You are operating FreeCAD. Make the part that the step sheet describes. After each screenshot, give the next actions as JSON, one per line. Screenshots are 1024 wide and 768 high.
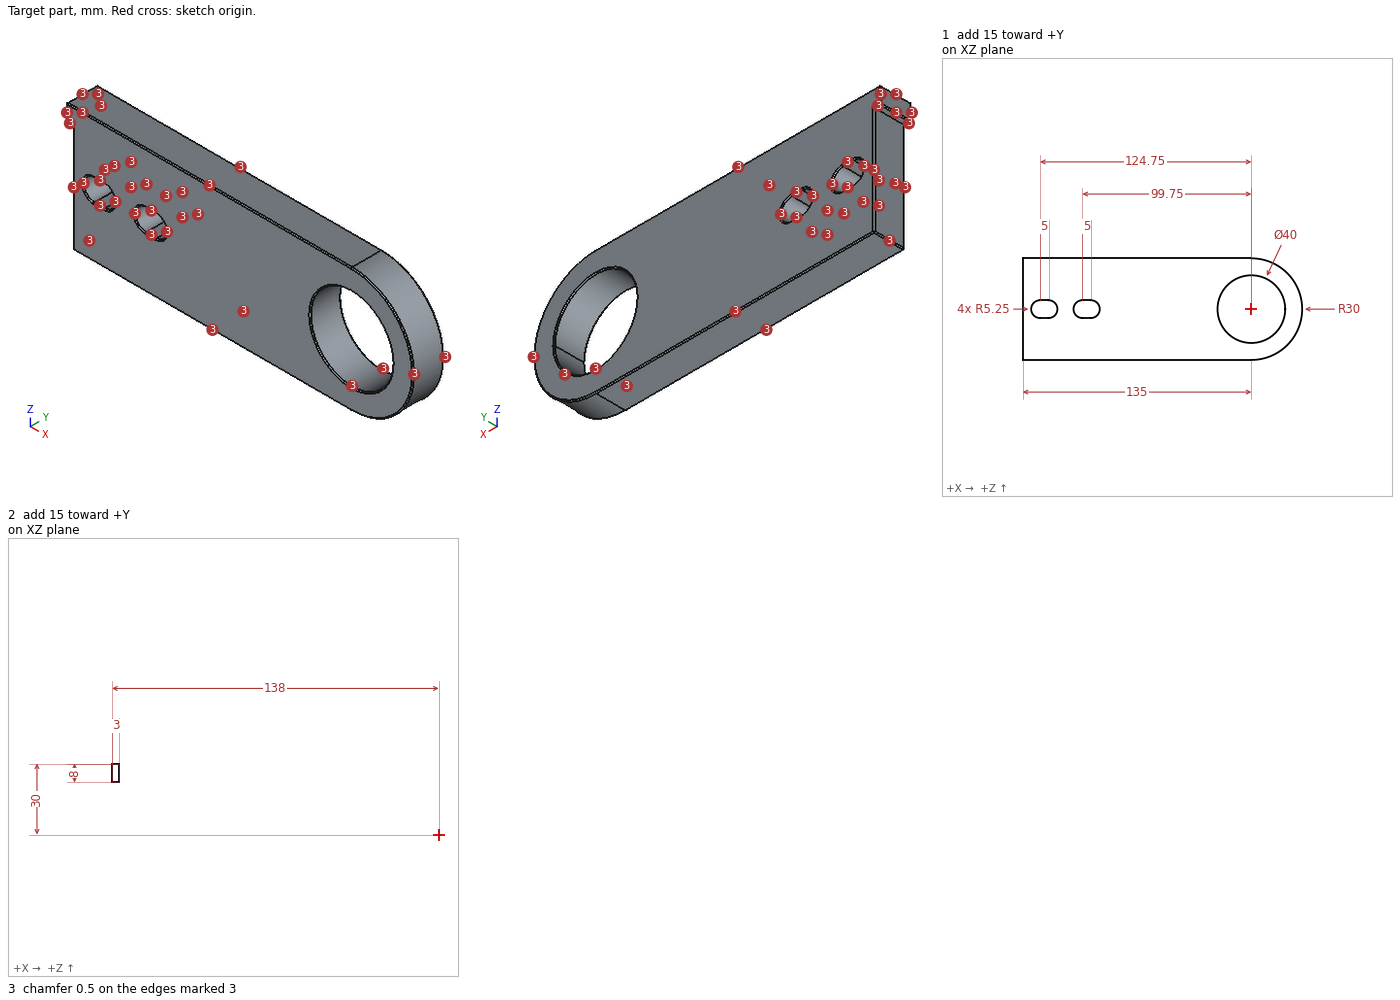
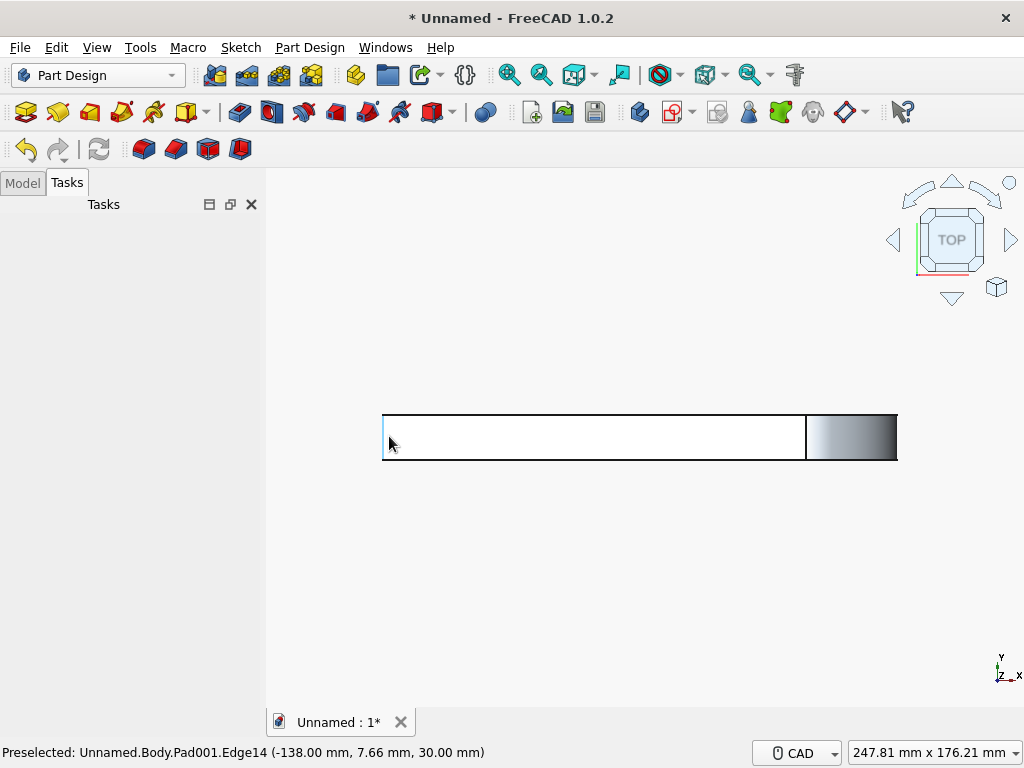
{"action": "key", "text": "1"}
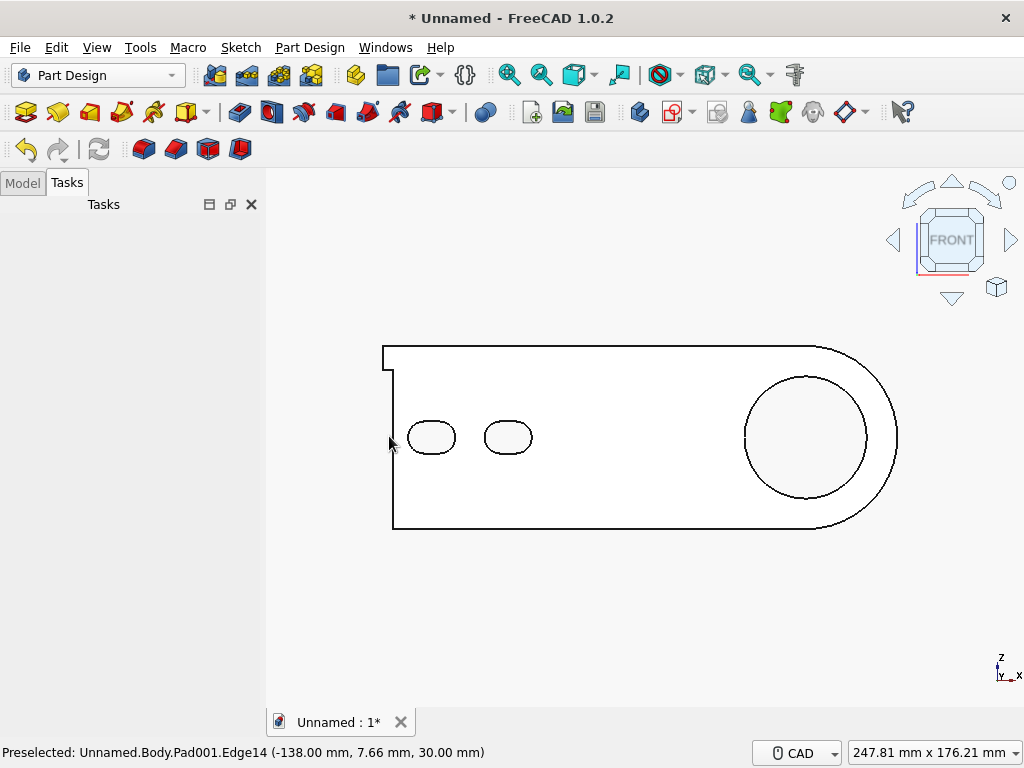
{"action": "key", "text": "3"}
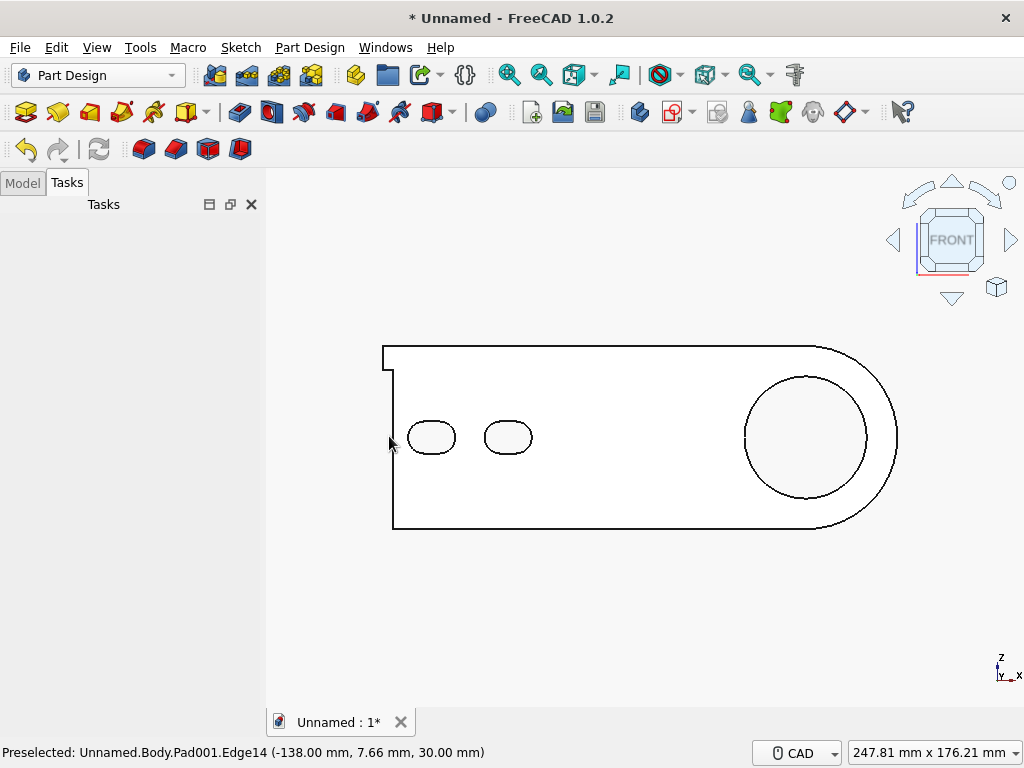
{"action": "left_click", "coordinate": [510, 76]}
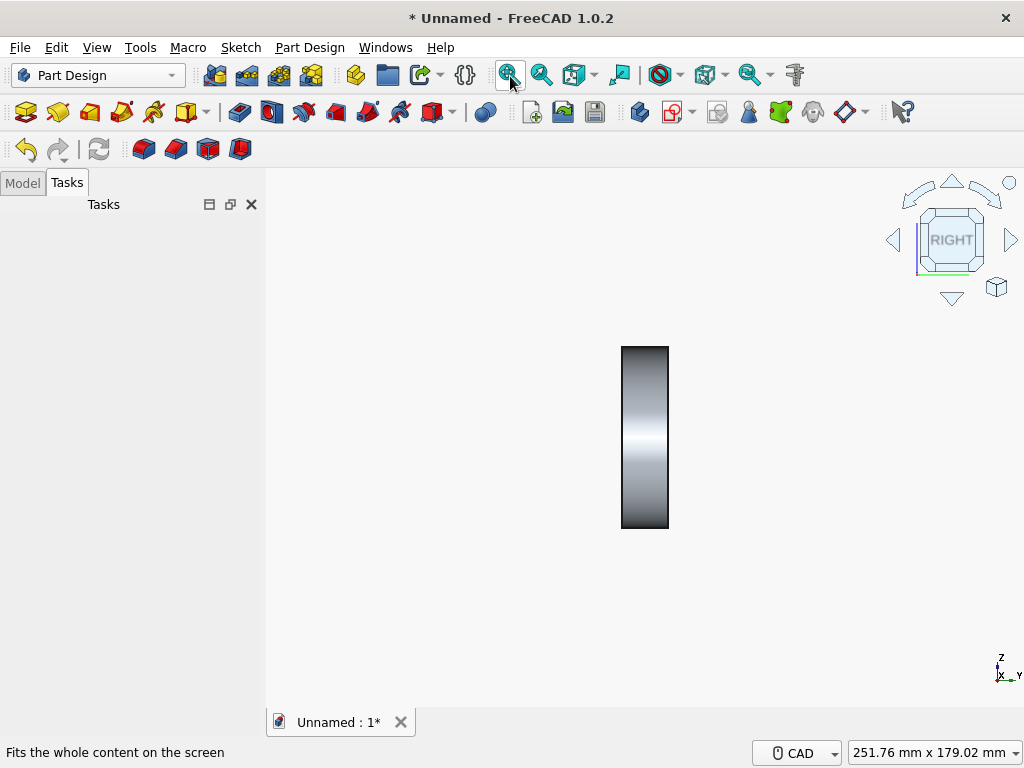
{"action": "key", "text": "5"}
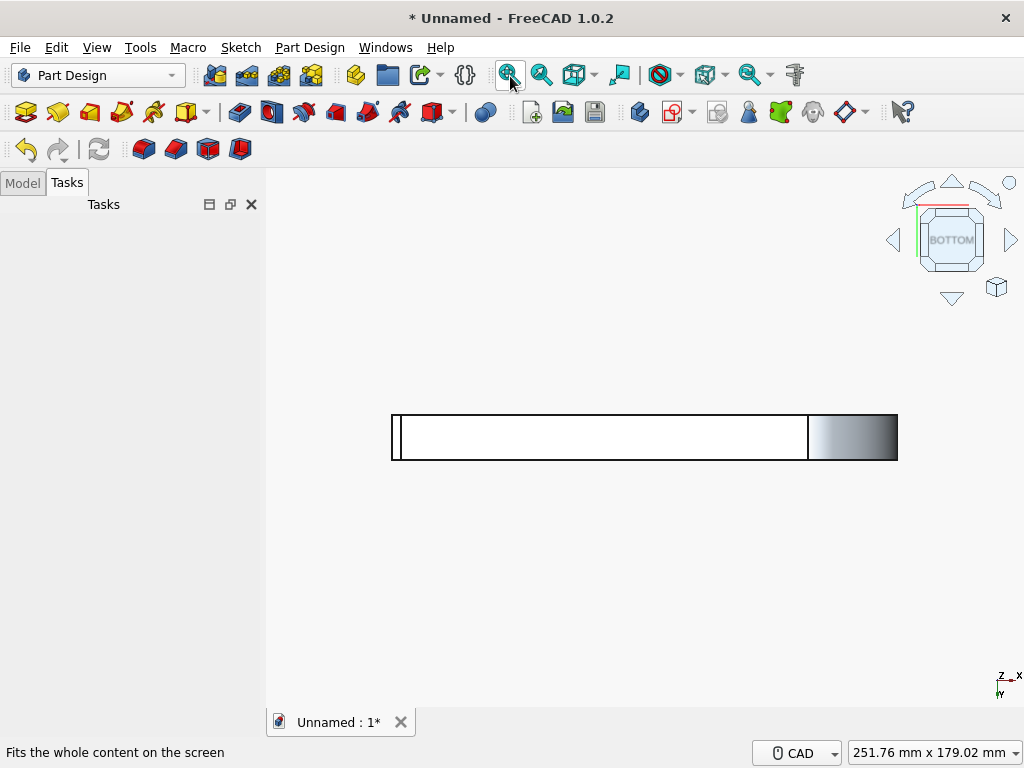
{"action": "left_click", "coordinate": [392, 436], "text": "ctrl"}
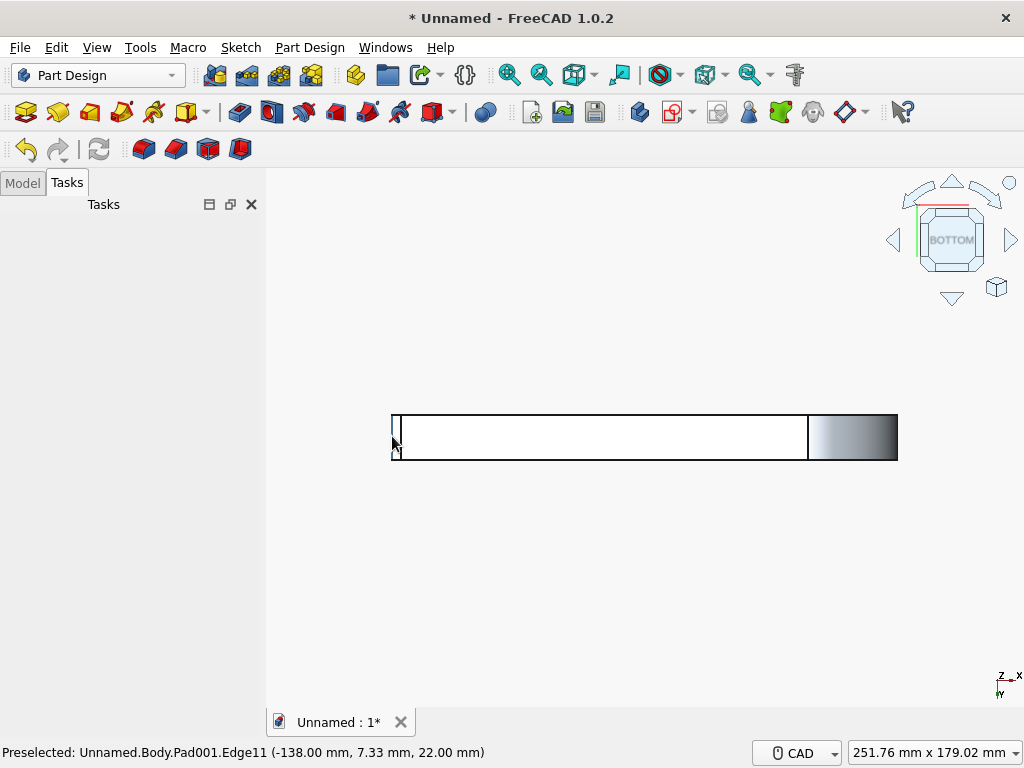
{"action": "left_click", "coordinate": [401, 436], "text": "ctrl"}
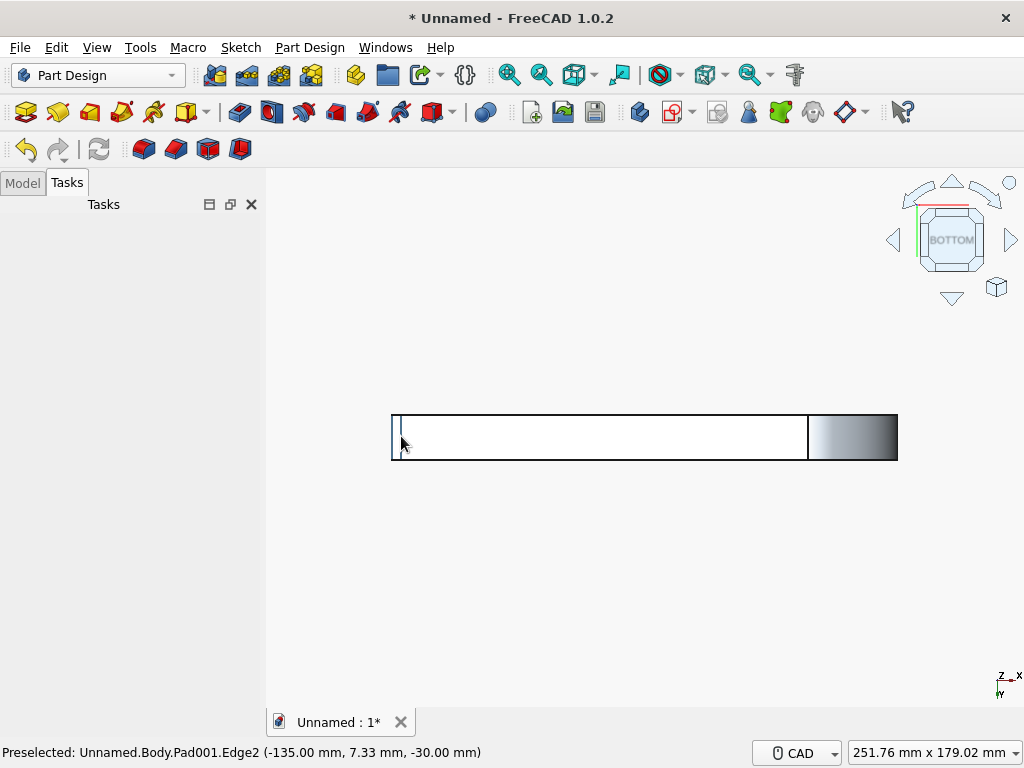
{"action": "key", "text": "4"}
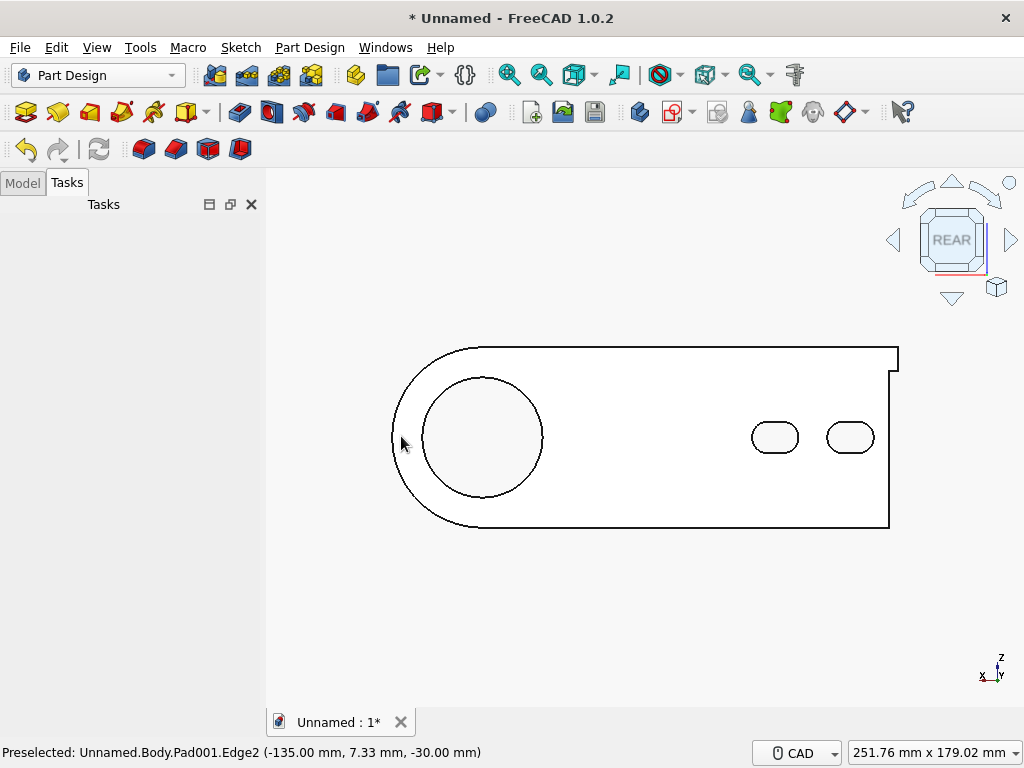
{"action": "left_click", "coordinate": [645, 437], "text": "ctrl"}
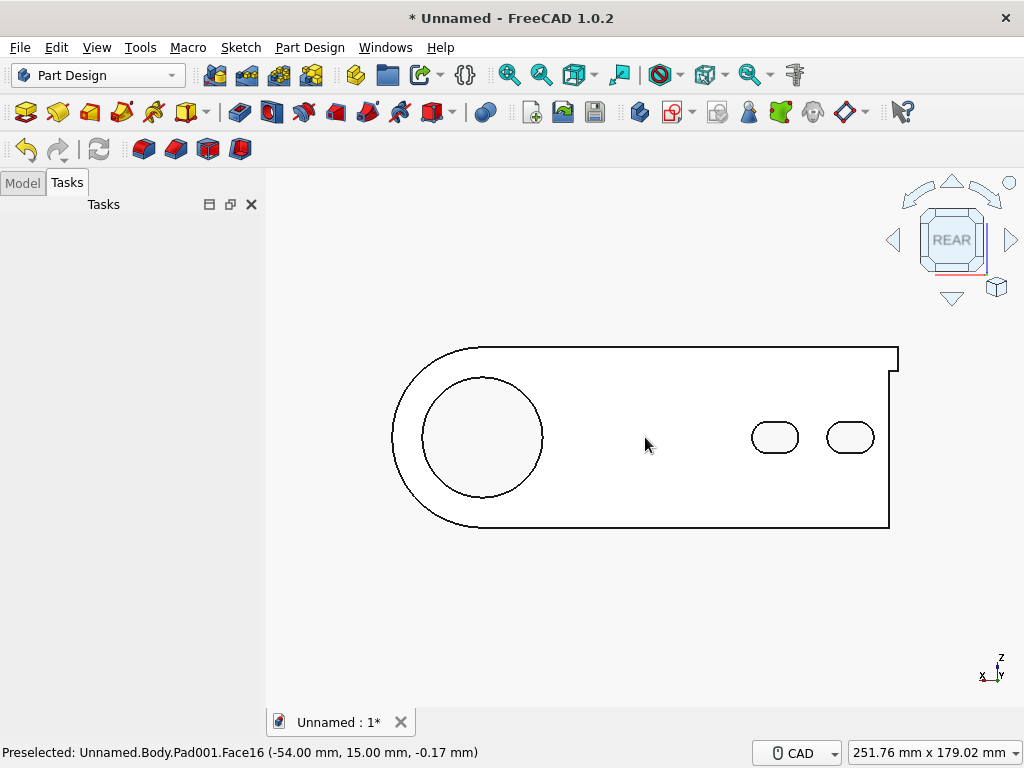
{"action": "left_click", "coordinate": [176, 150]}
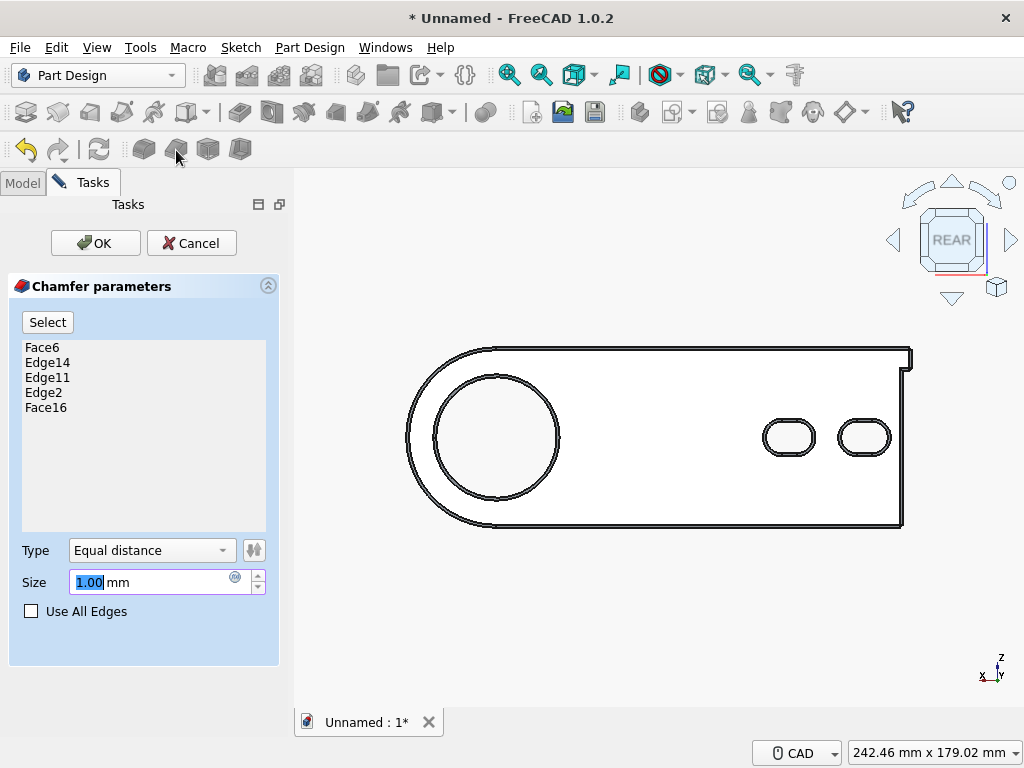
{"action": "type", "text": "0.5"}
{"action": "key", "text": "Tab"}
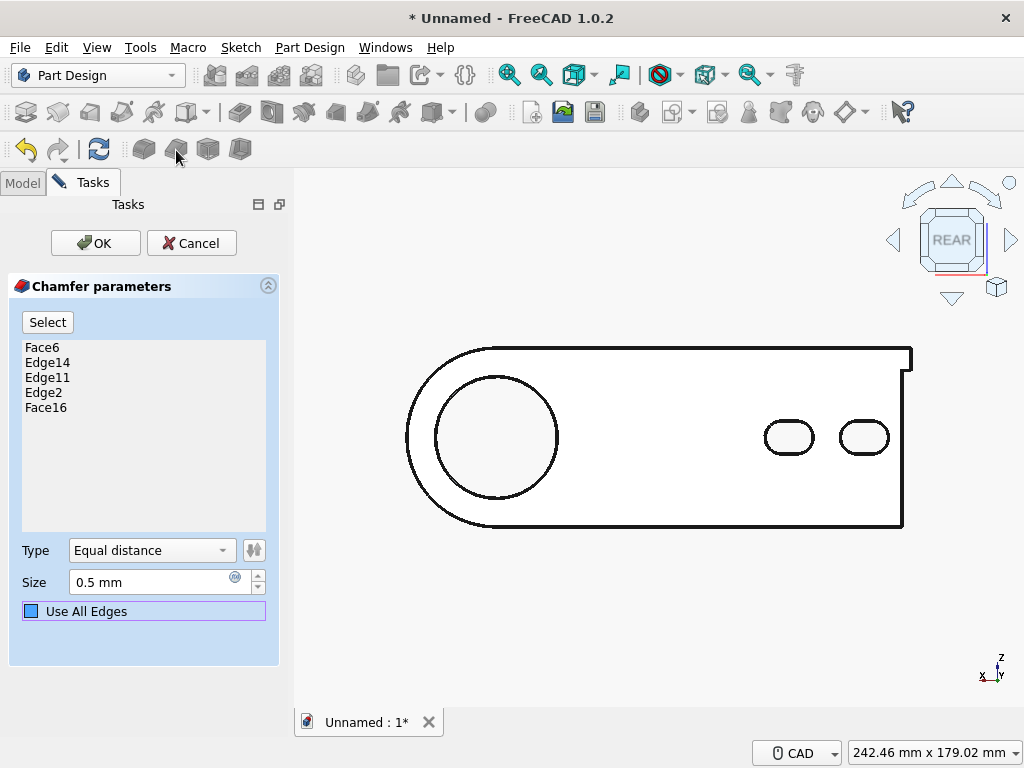
{"action": "left_click", "coordinate": [96, 243]}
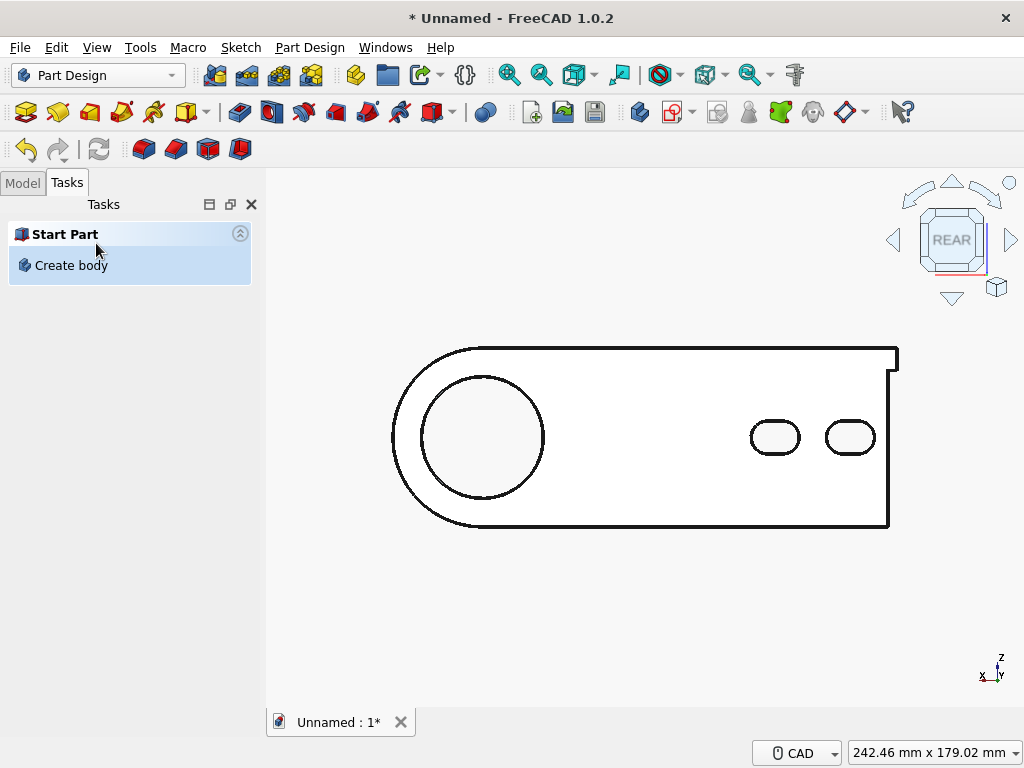
{"action": "key", "text": "0"}